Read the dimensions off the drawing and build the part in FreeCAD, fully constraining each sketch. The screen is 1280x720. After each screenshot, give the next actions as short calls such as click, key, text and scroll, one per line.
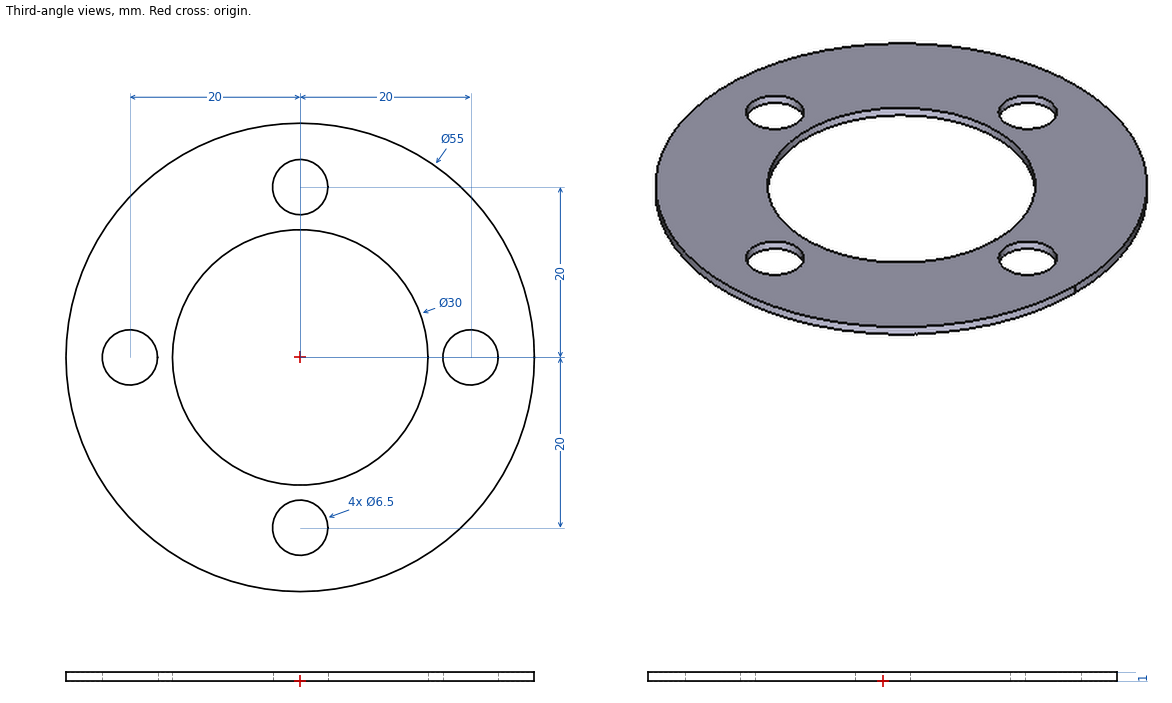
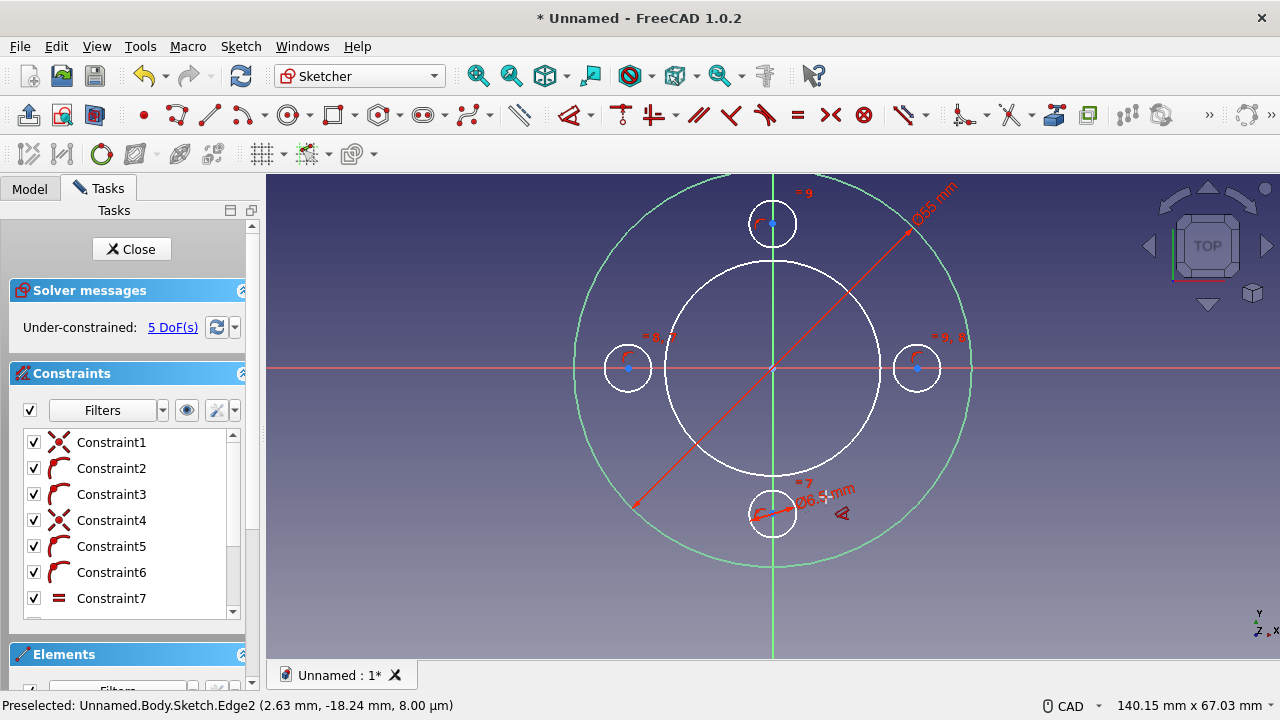
click(849, 292)
click(872, 269)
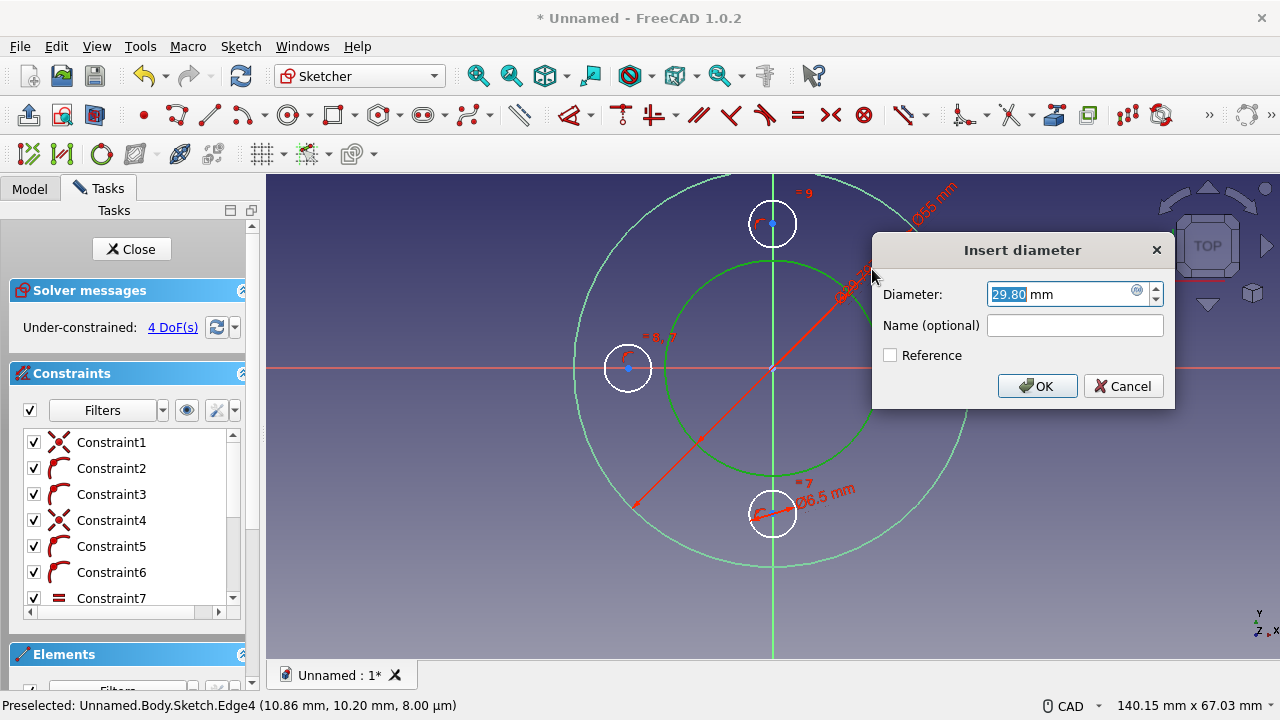
text(30)
key(Return)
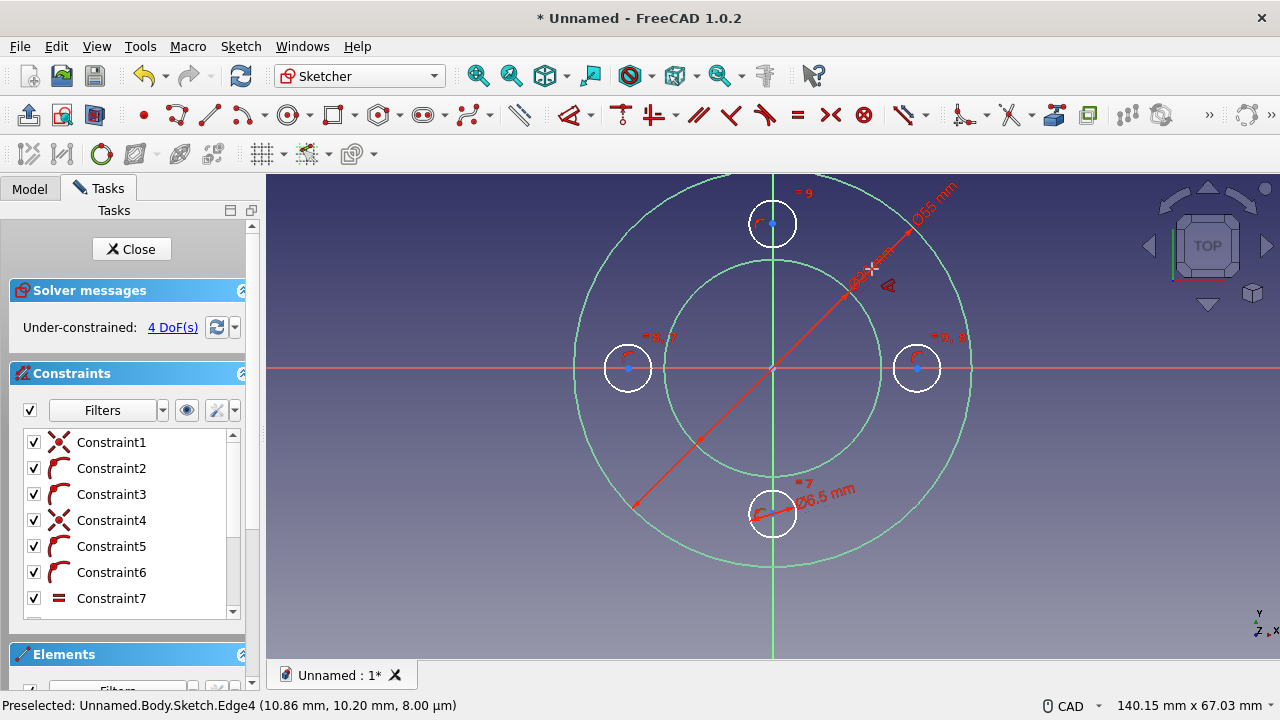
click(773, 514)
click(807, 441)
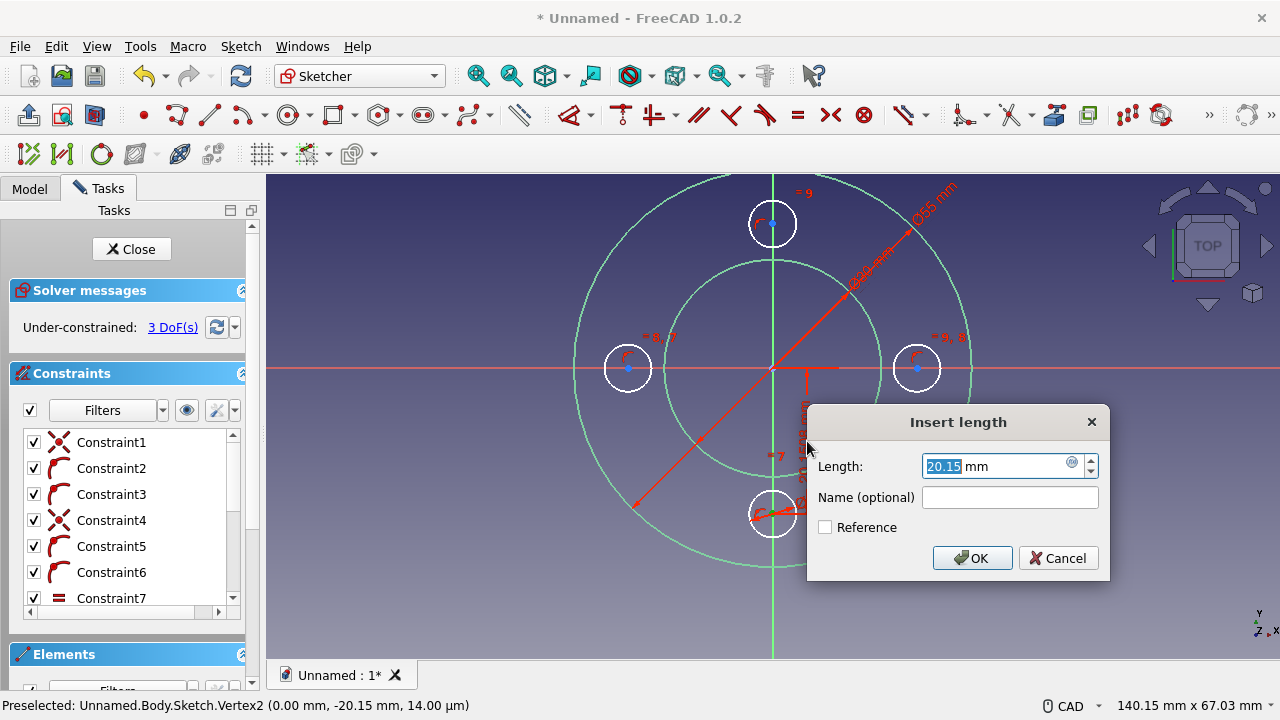
text(20)
key(Return)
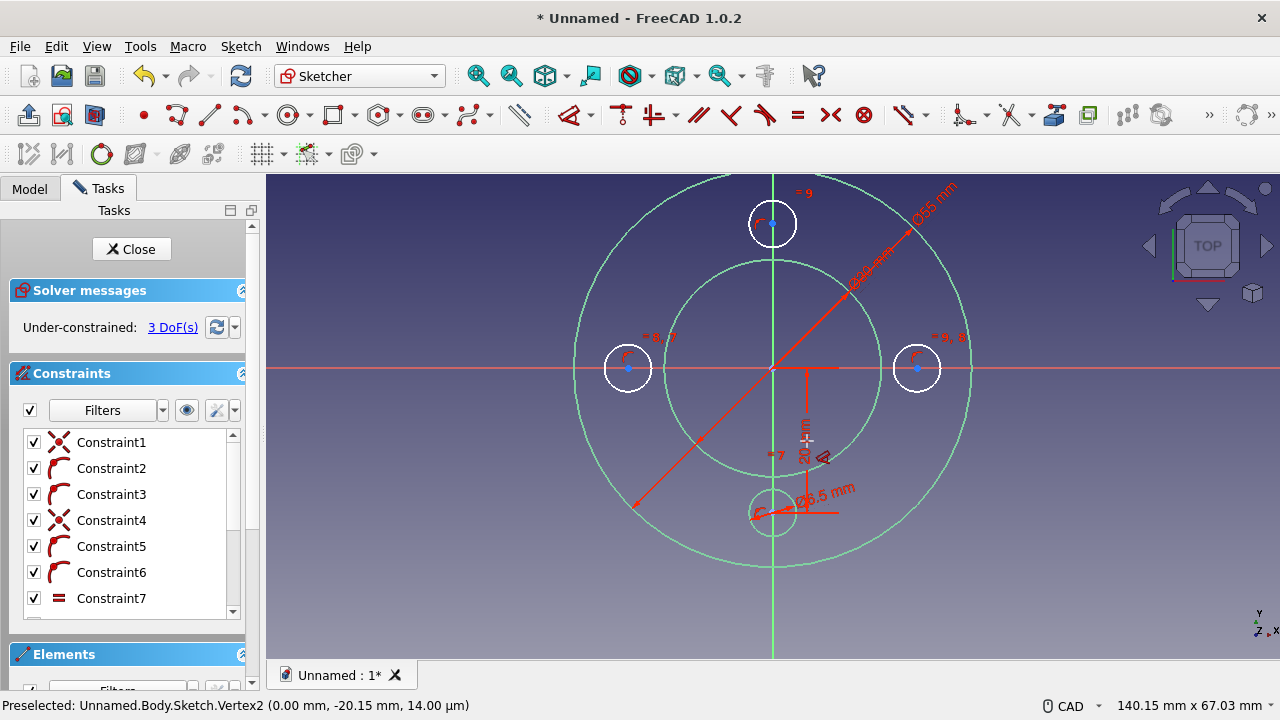
click(628, 368)
click(700, 402)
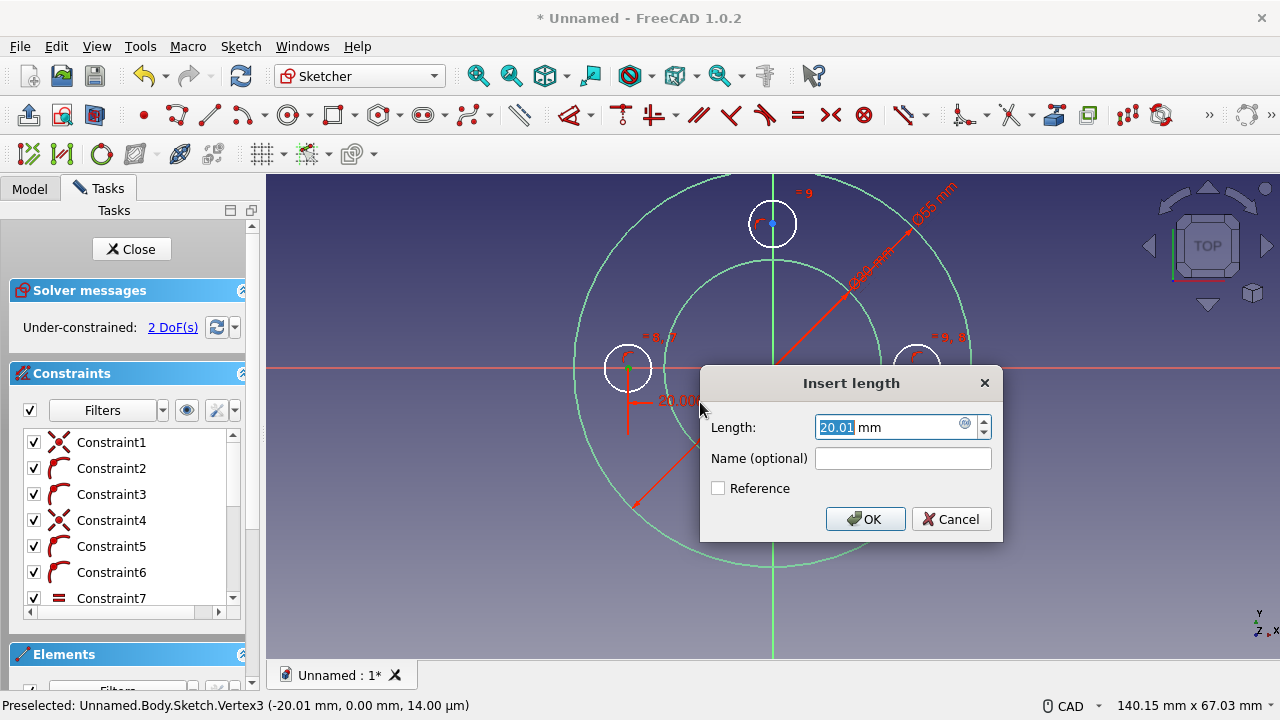
text(20)
key(Return)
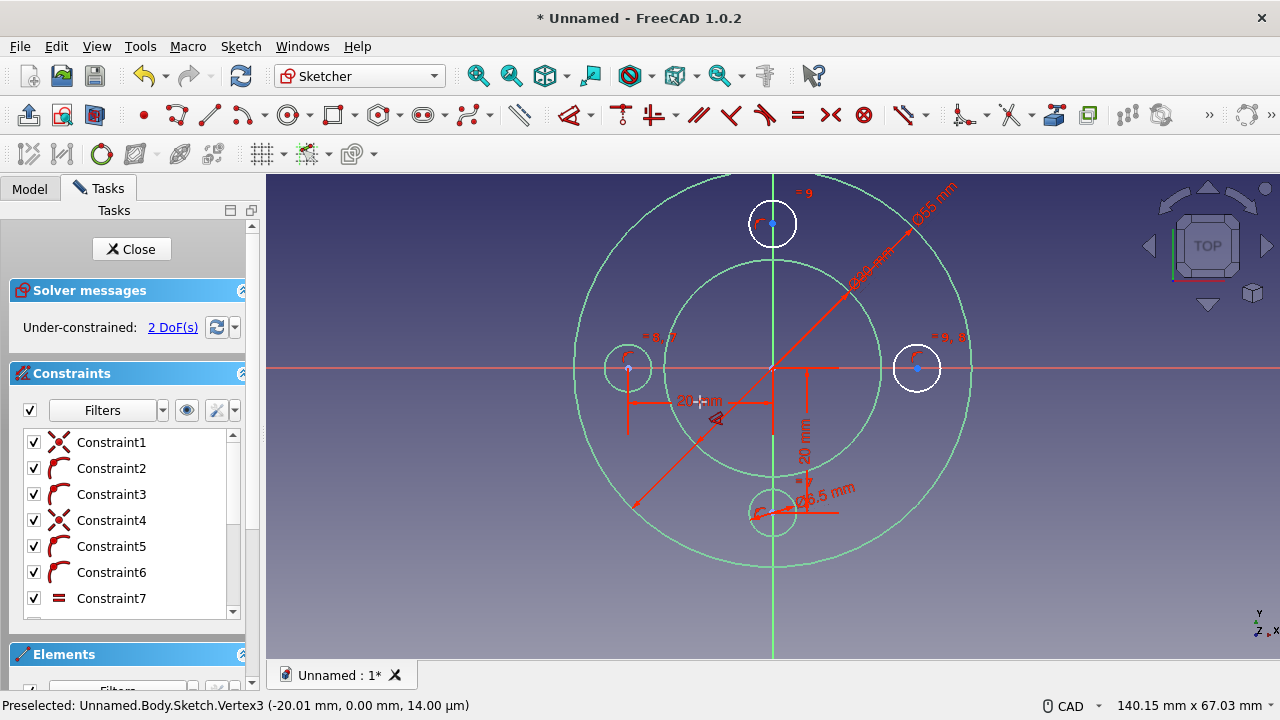
click(917, 368)
click(845, 402)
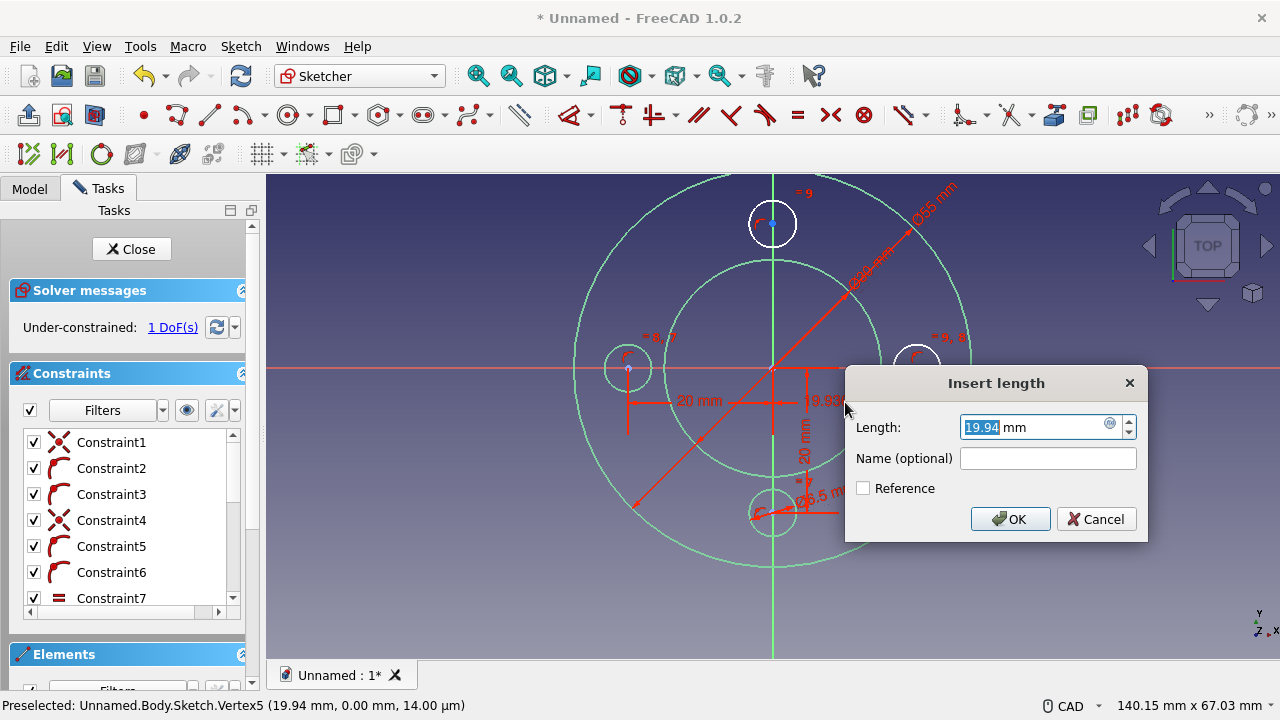
text(20)
key(Return)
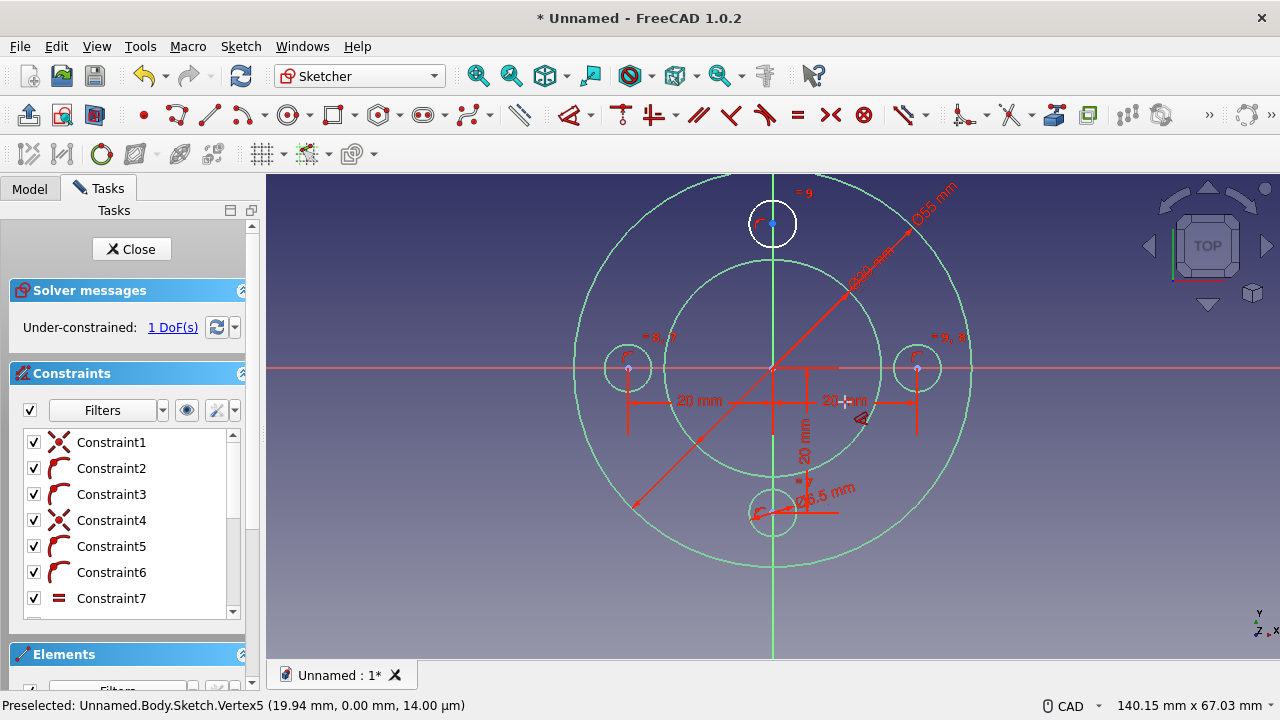
click(773, 224)
click(807, 296)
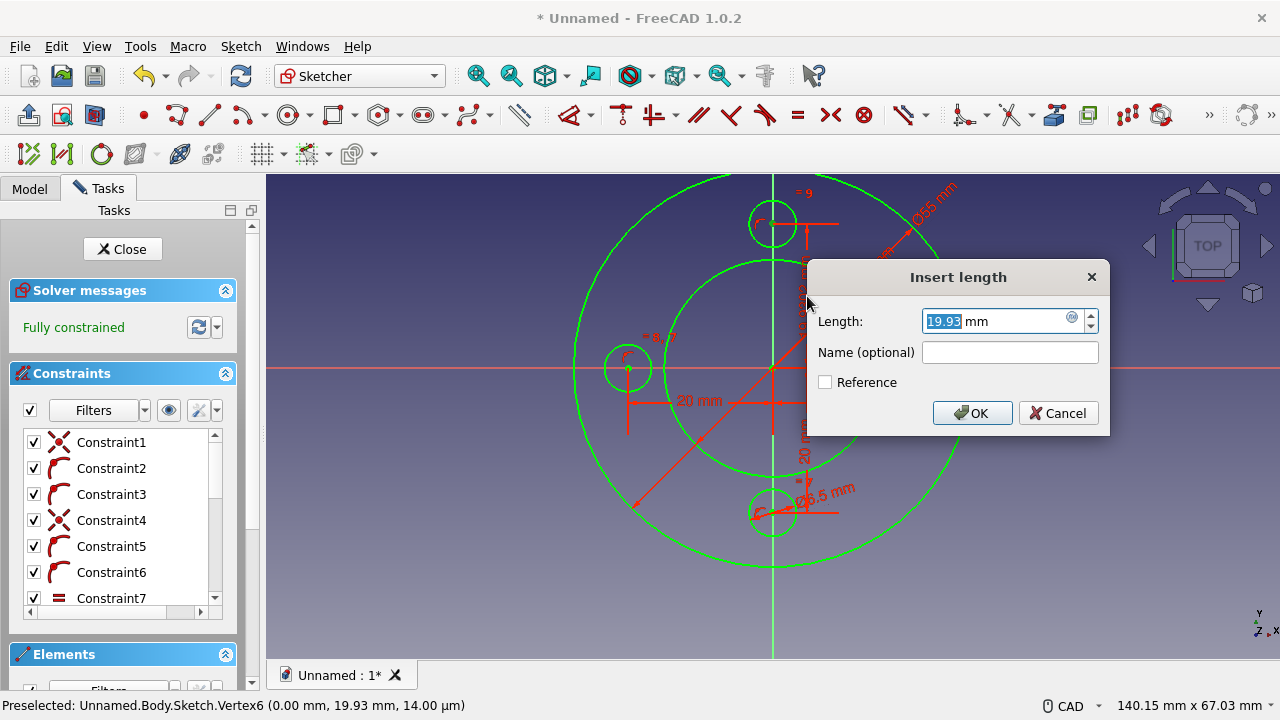
text(20)
key(Return)
key(Escape)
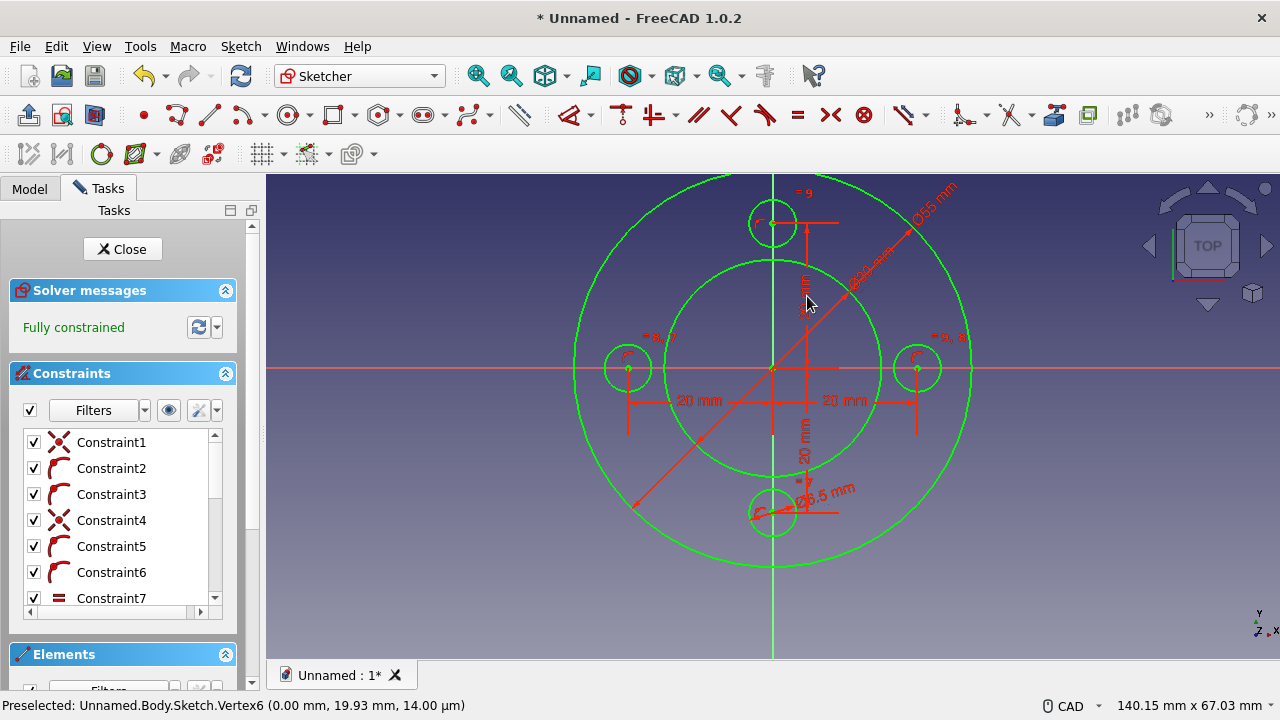
click(123, 249)